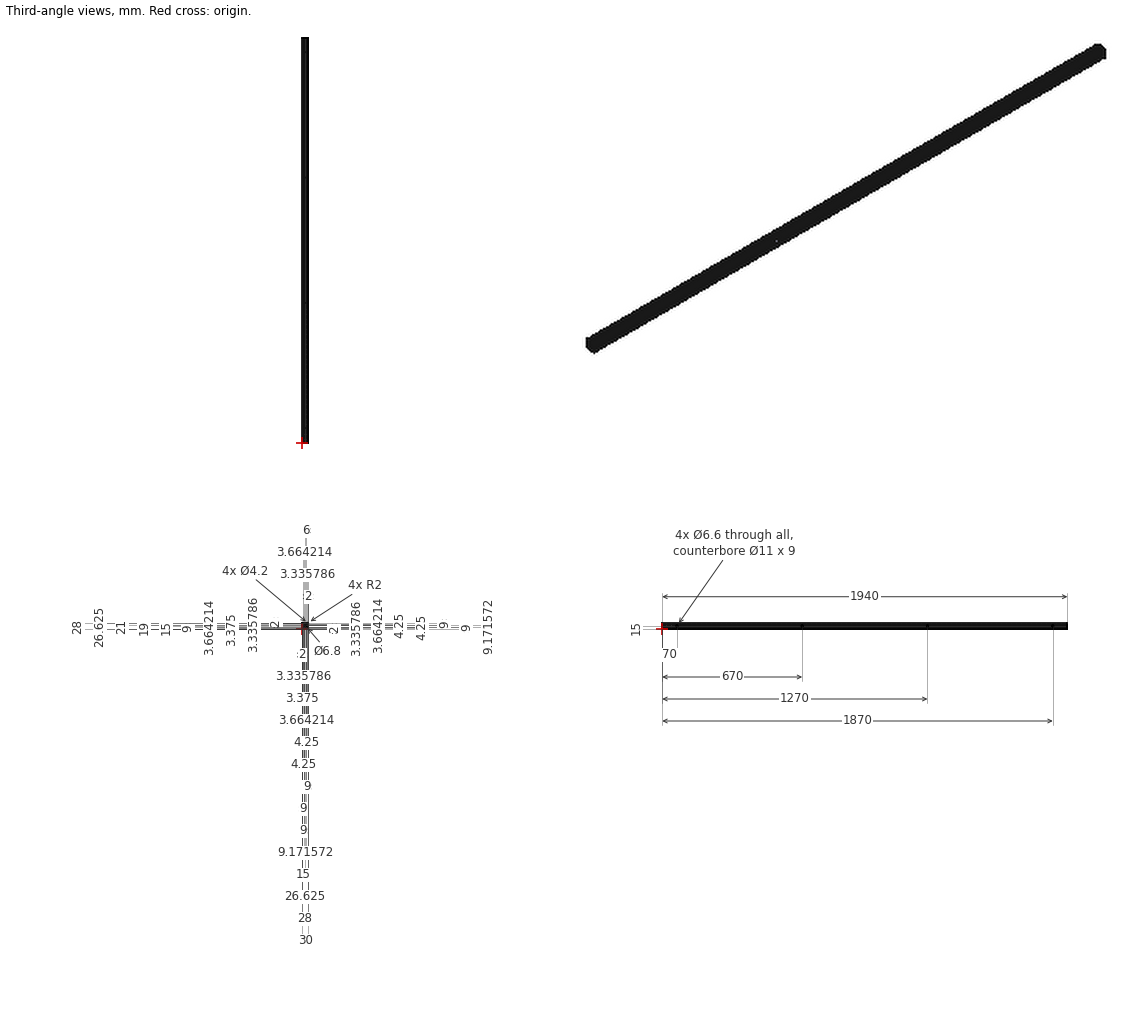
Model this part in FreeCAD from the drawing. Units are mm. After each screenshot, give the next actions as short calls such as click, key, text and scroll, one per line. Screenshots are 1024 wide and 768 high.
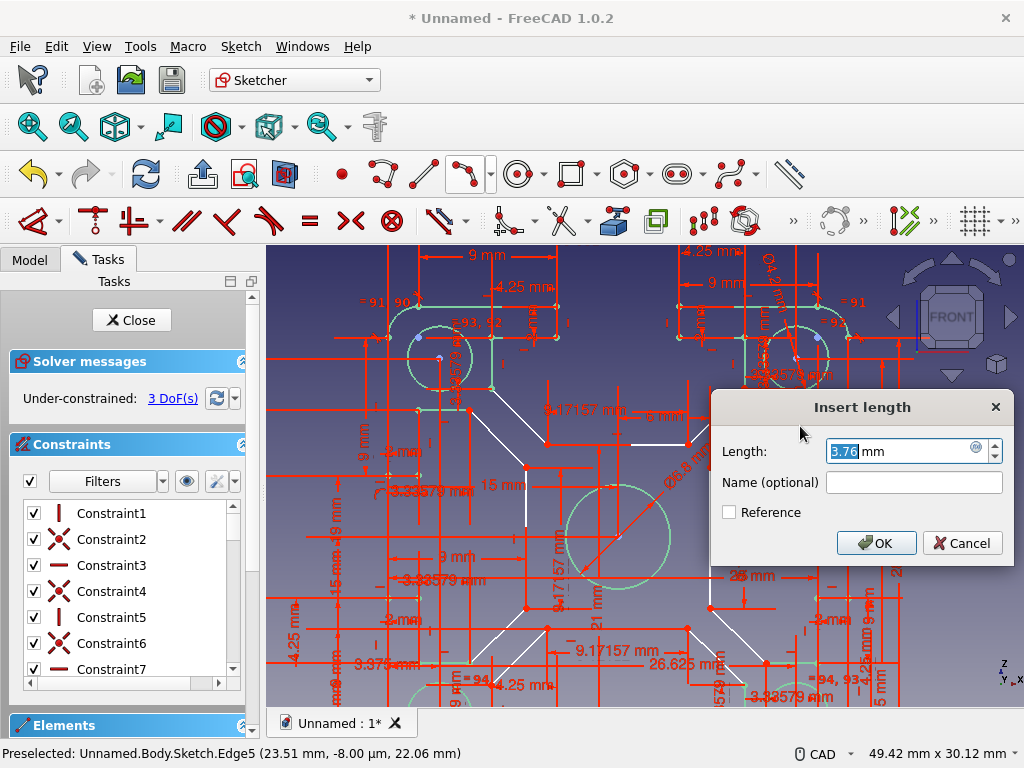
text(3.664214)
key(Return)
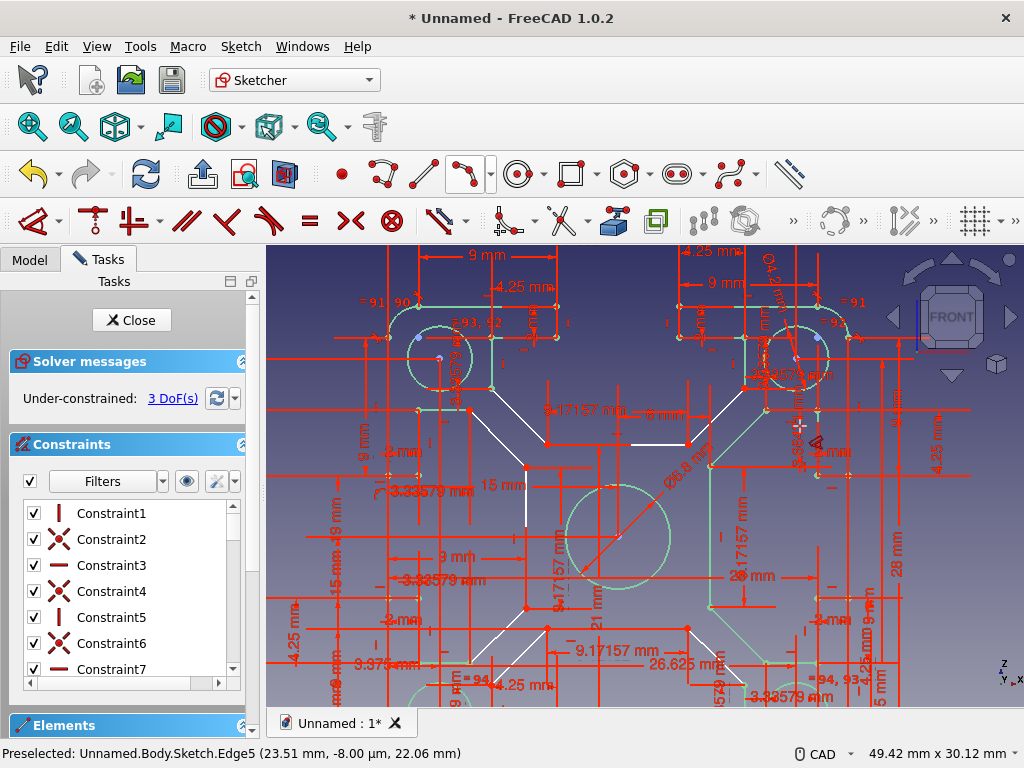
click(728, 668)
click(729, 499)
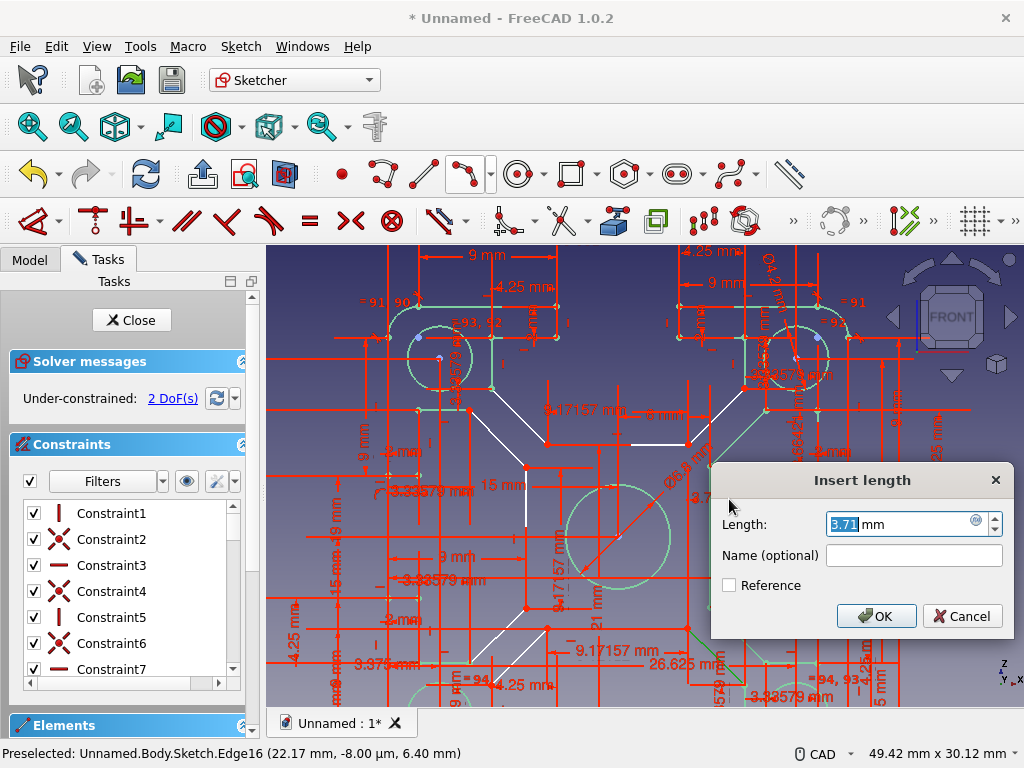
text(3.664214)
key(Return)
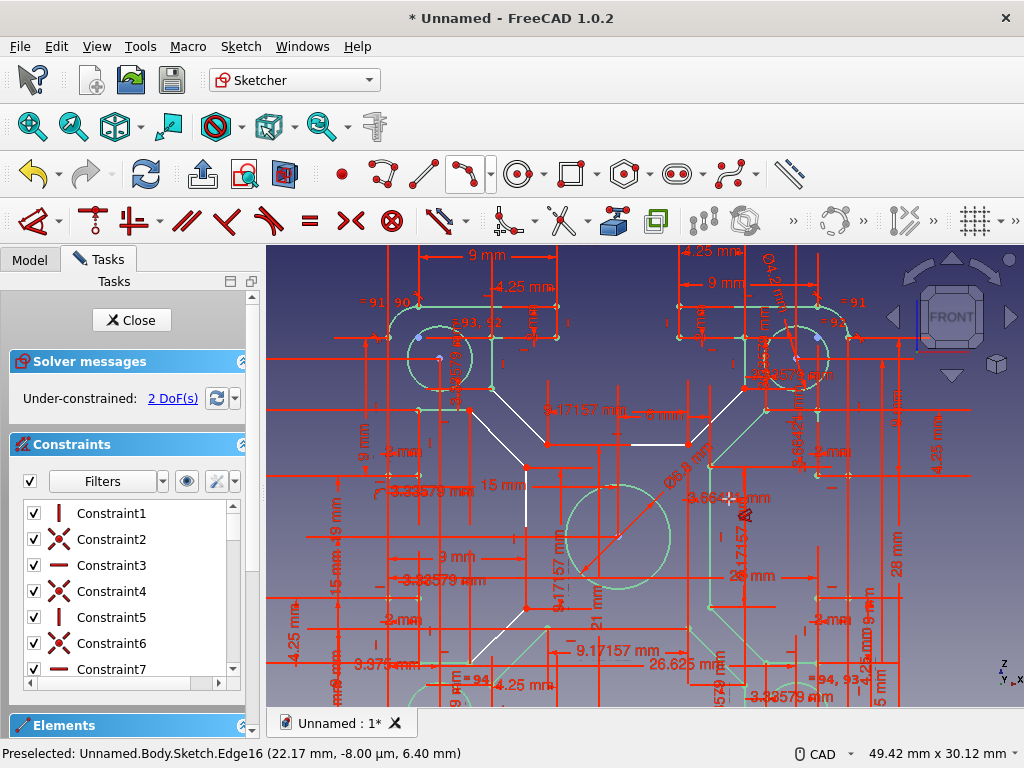
click(487, 647)
click(706, 623)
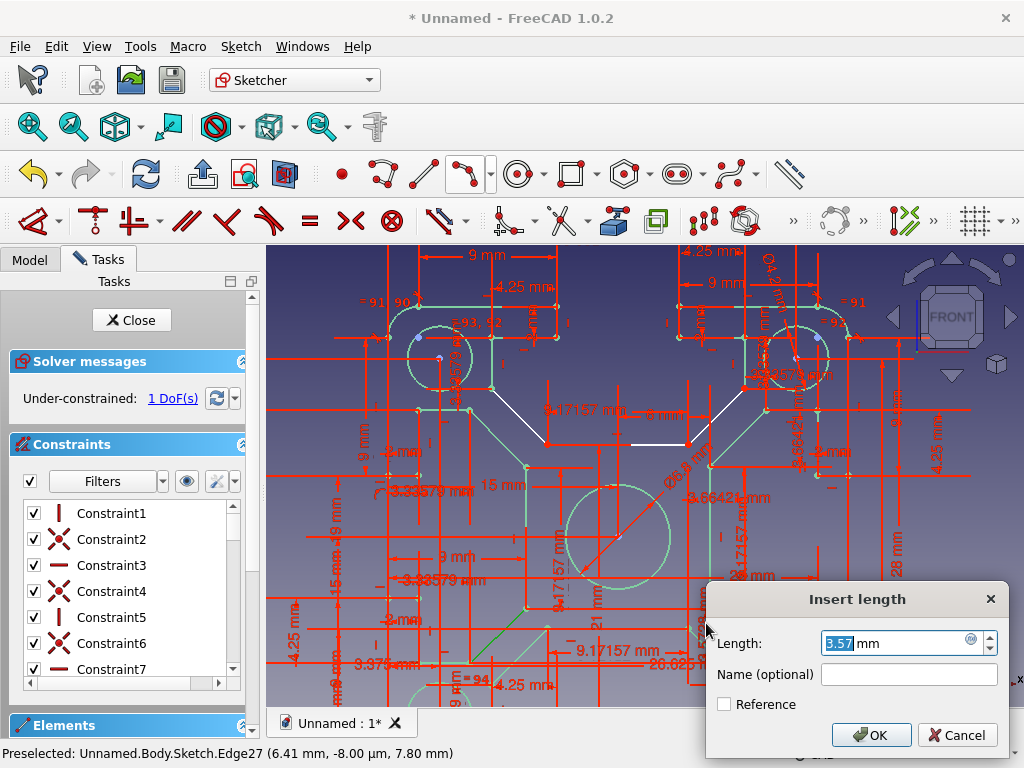
text(3.664214)
key(Return)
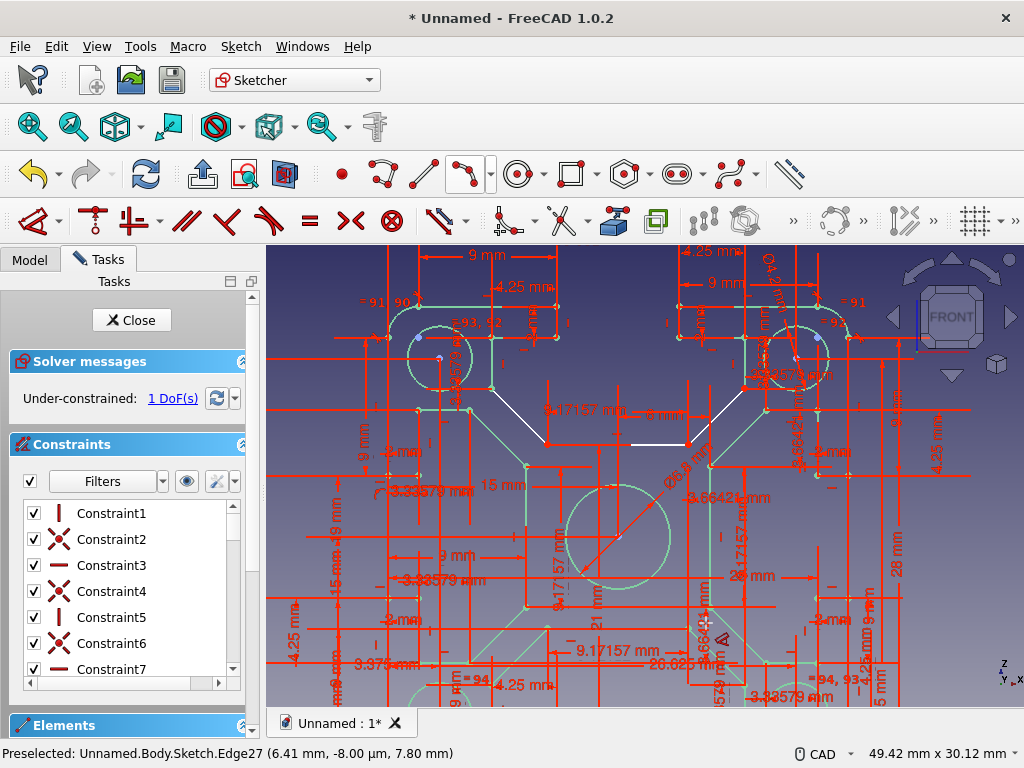
click(508, 406)
click(532, 355)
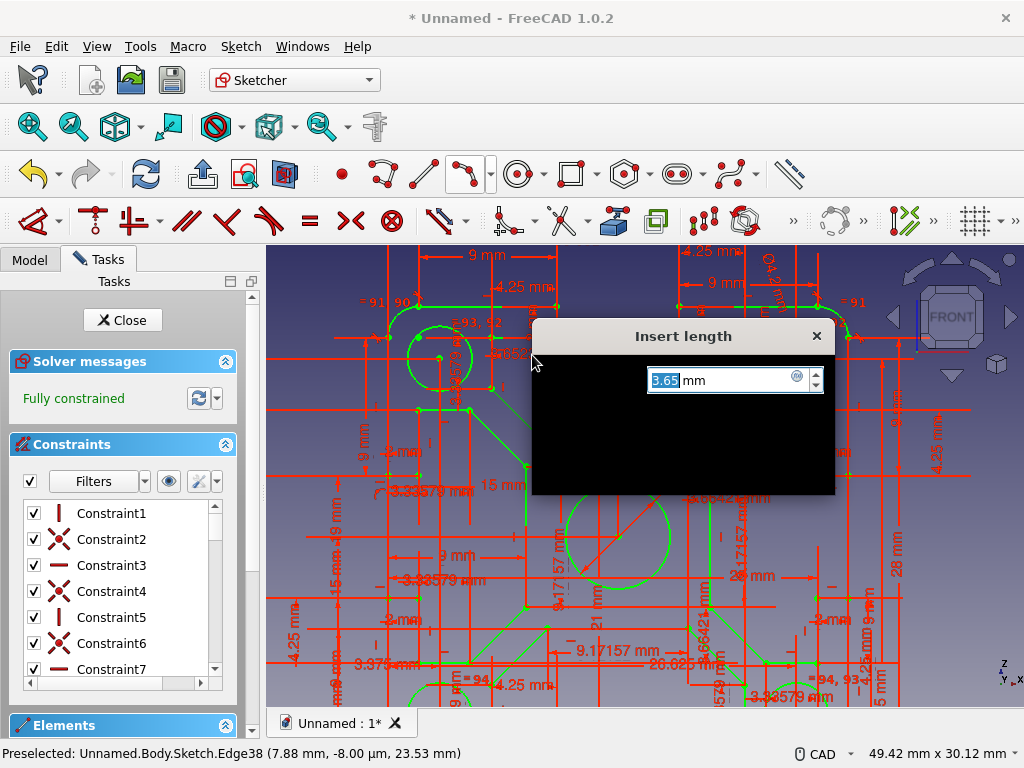
text(3.664214)
key(Return)
key(Escape)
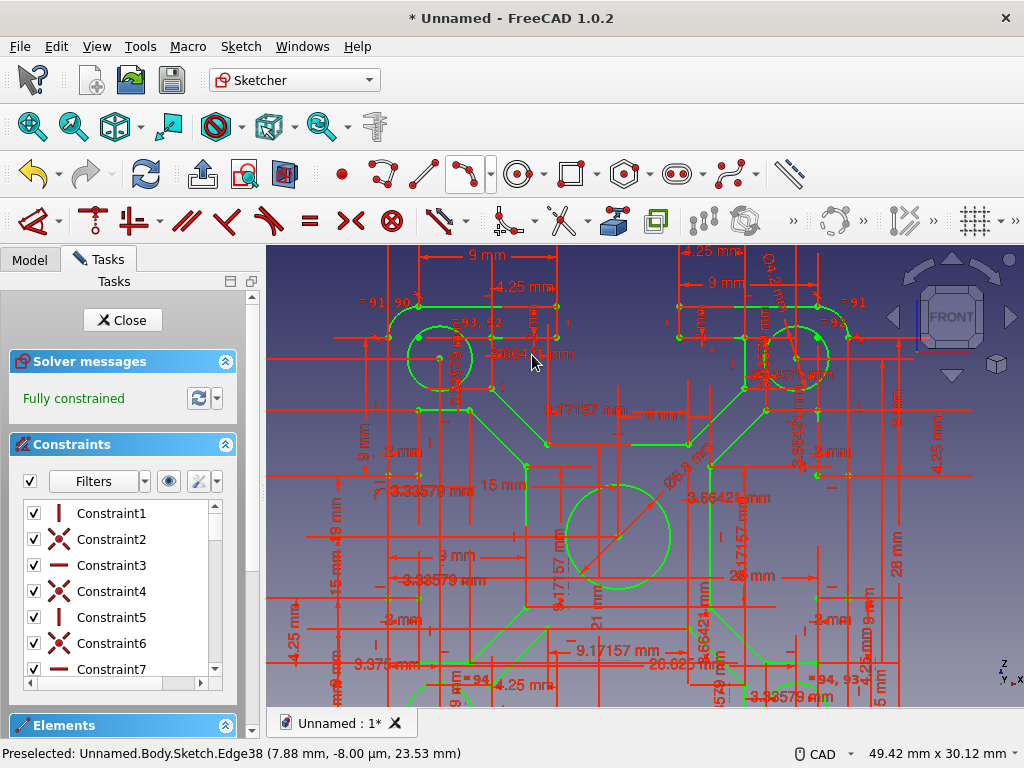
click(123, 320)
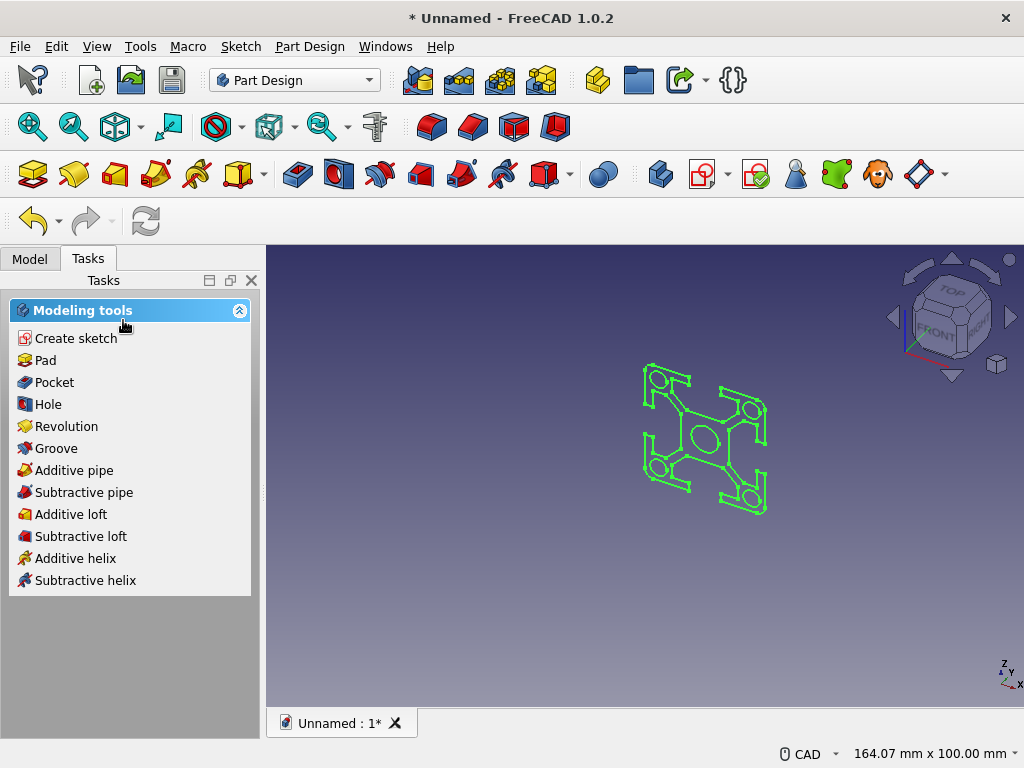
click(33, 174)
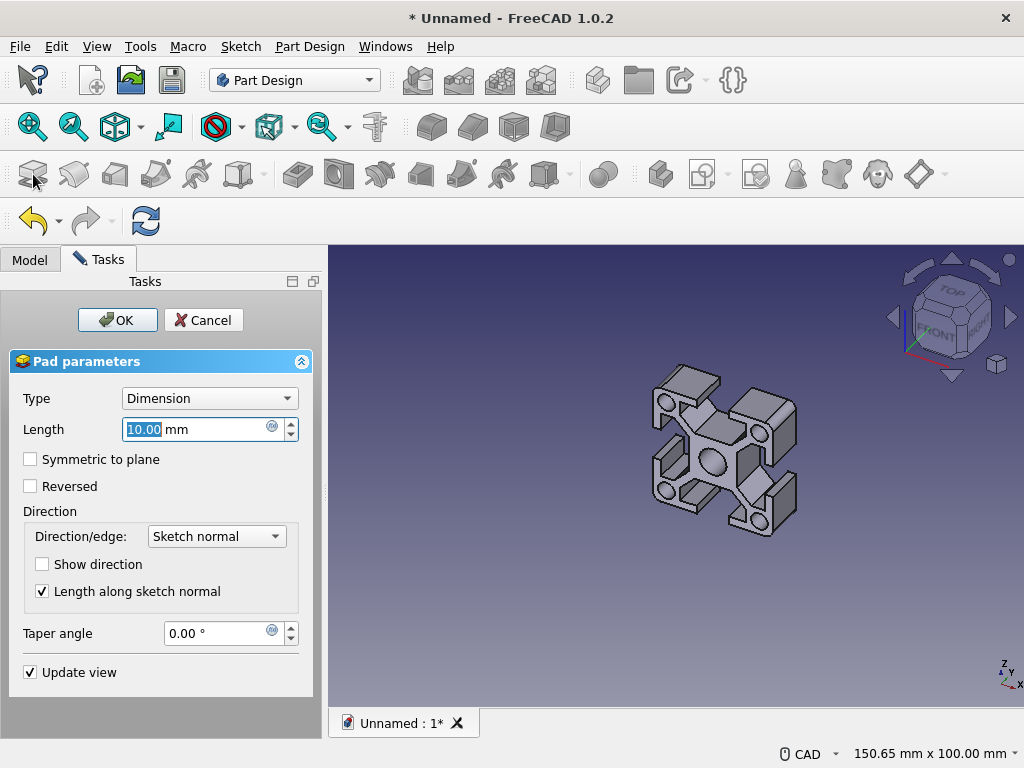
text(1940)
key(Tab)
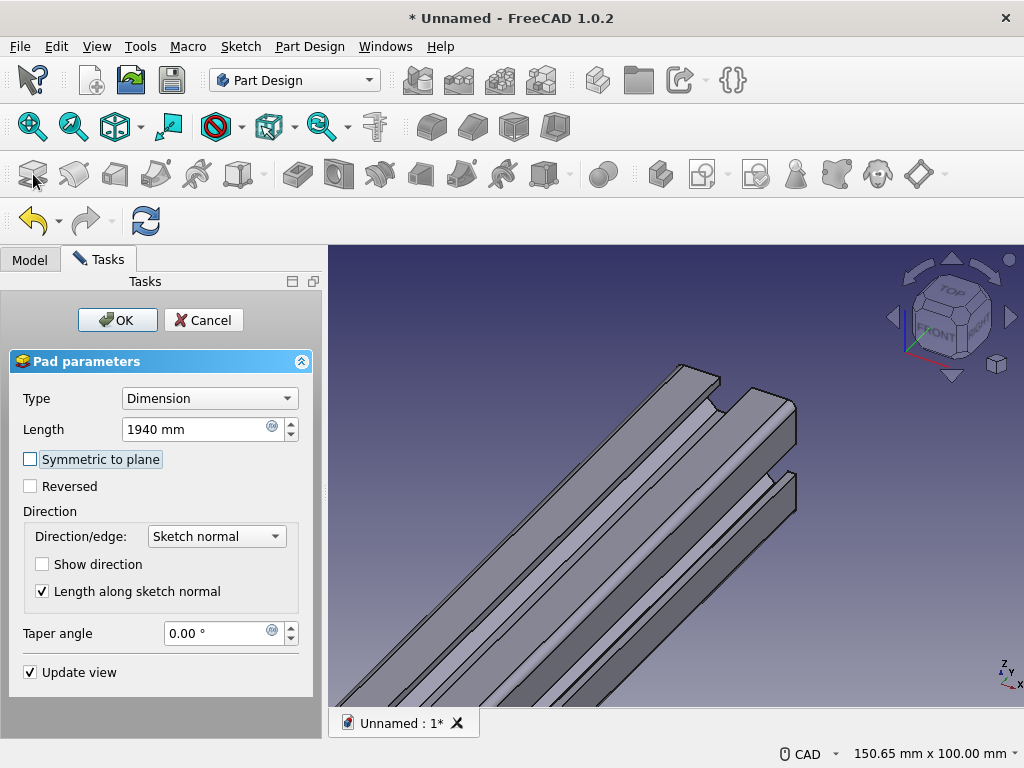
click(31, 486)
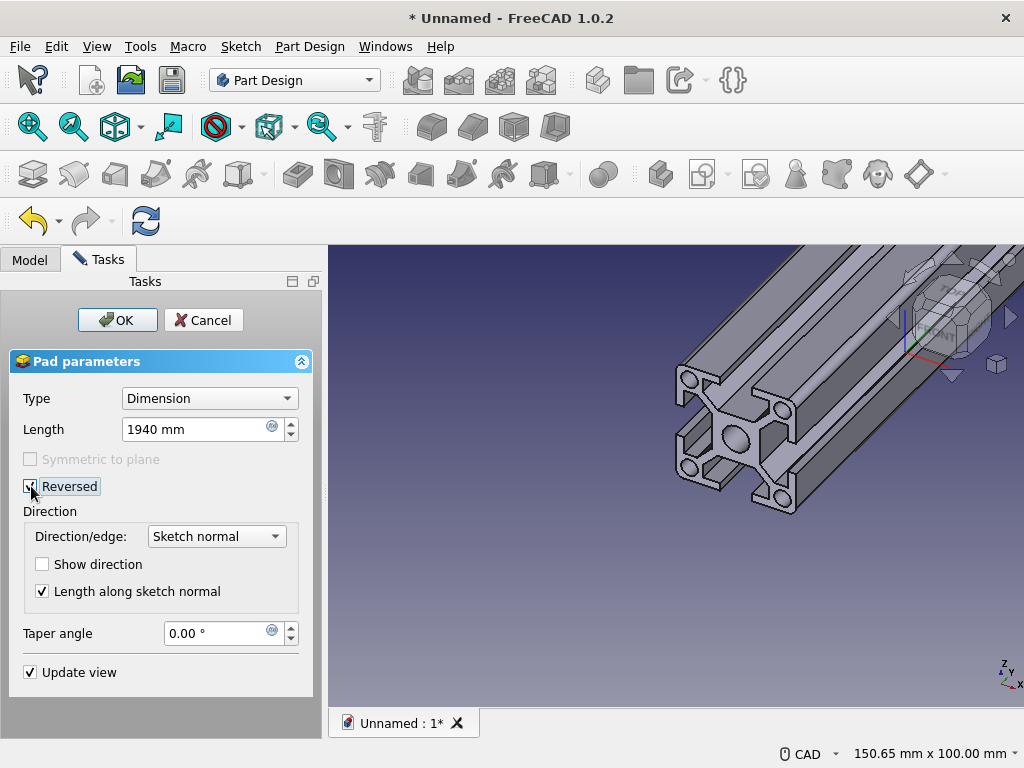
click(118, 320)